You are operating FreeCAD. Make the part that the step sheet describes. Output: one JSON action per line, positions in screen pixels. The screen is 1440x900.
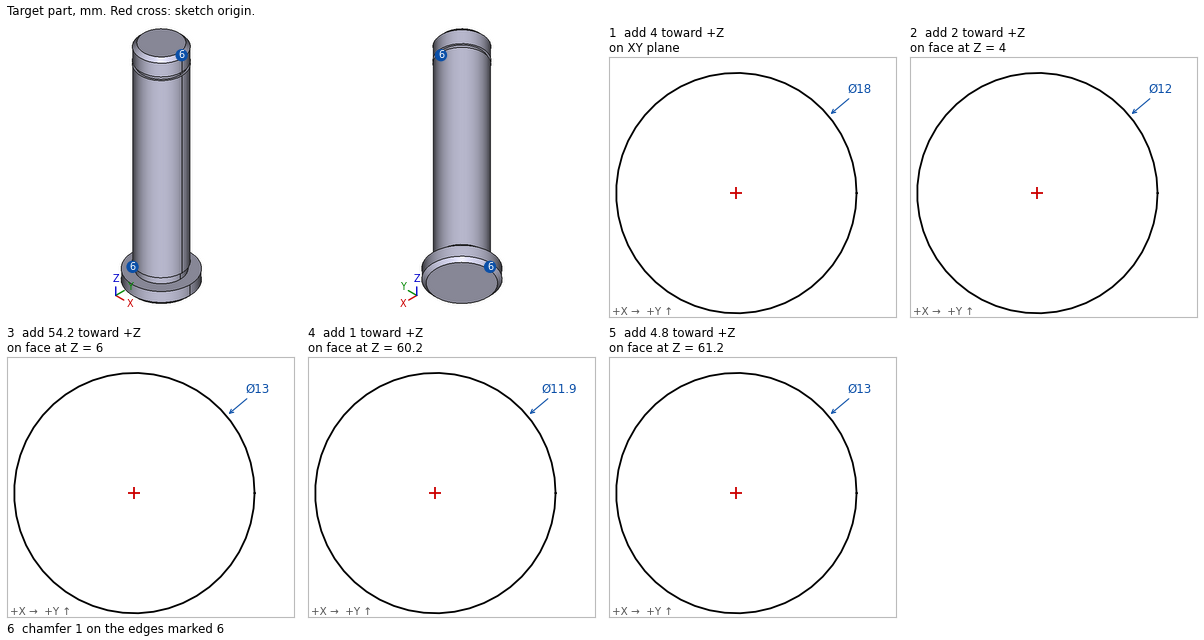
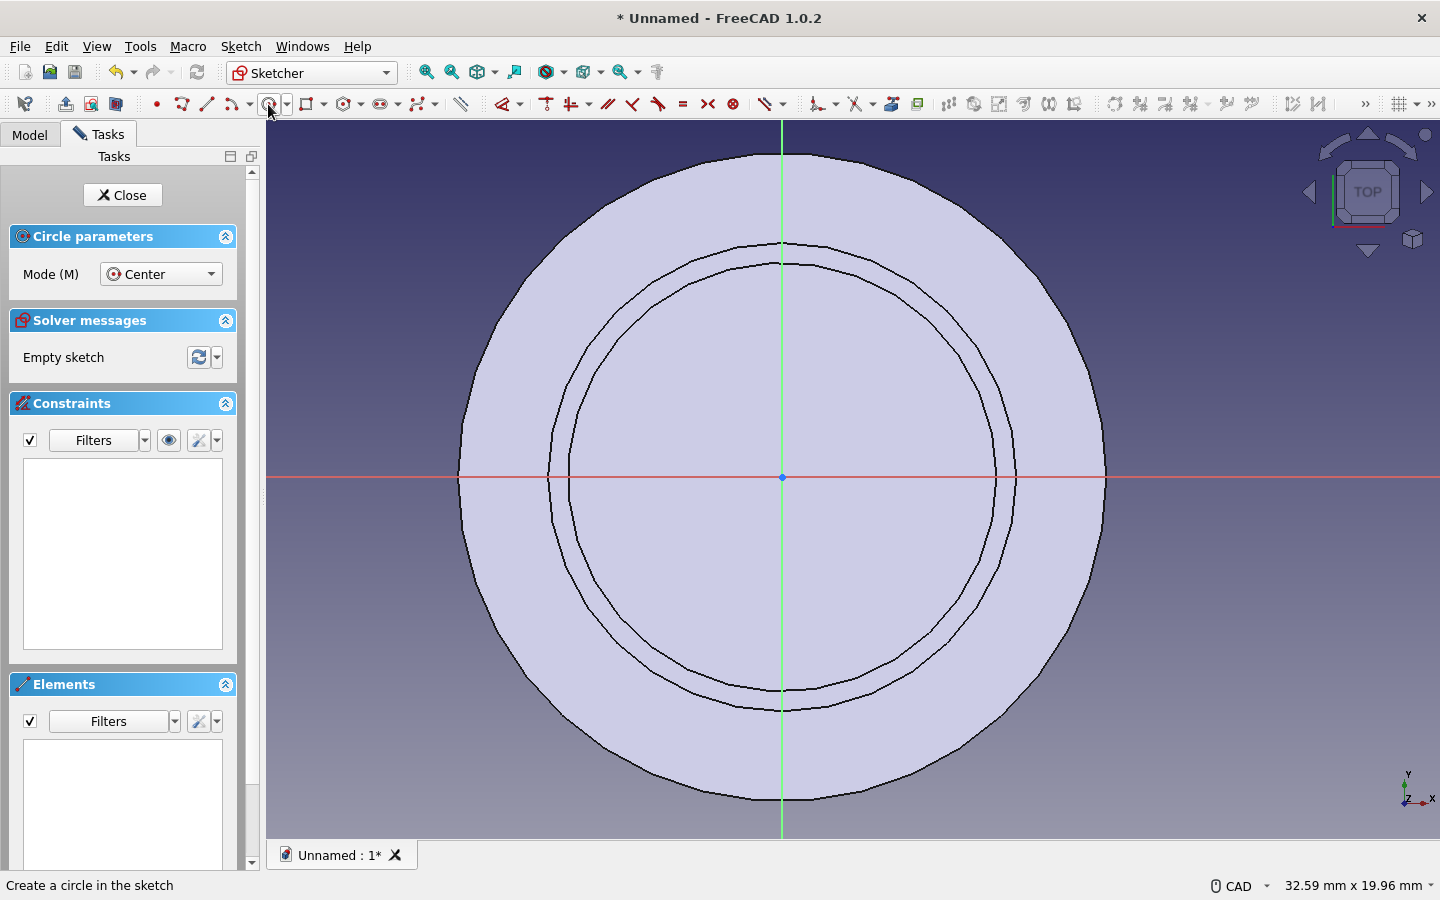
{"action": "left_click", "coordinate": [782, 477]}
{"action": "left_click", "coordinate": [948, 312]}
{"action": "key", "text": "Escape"}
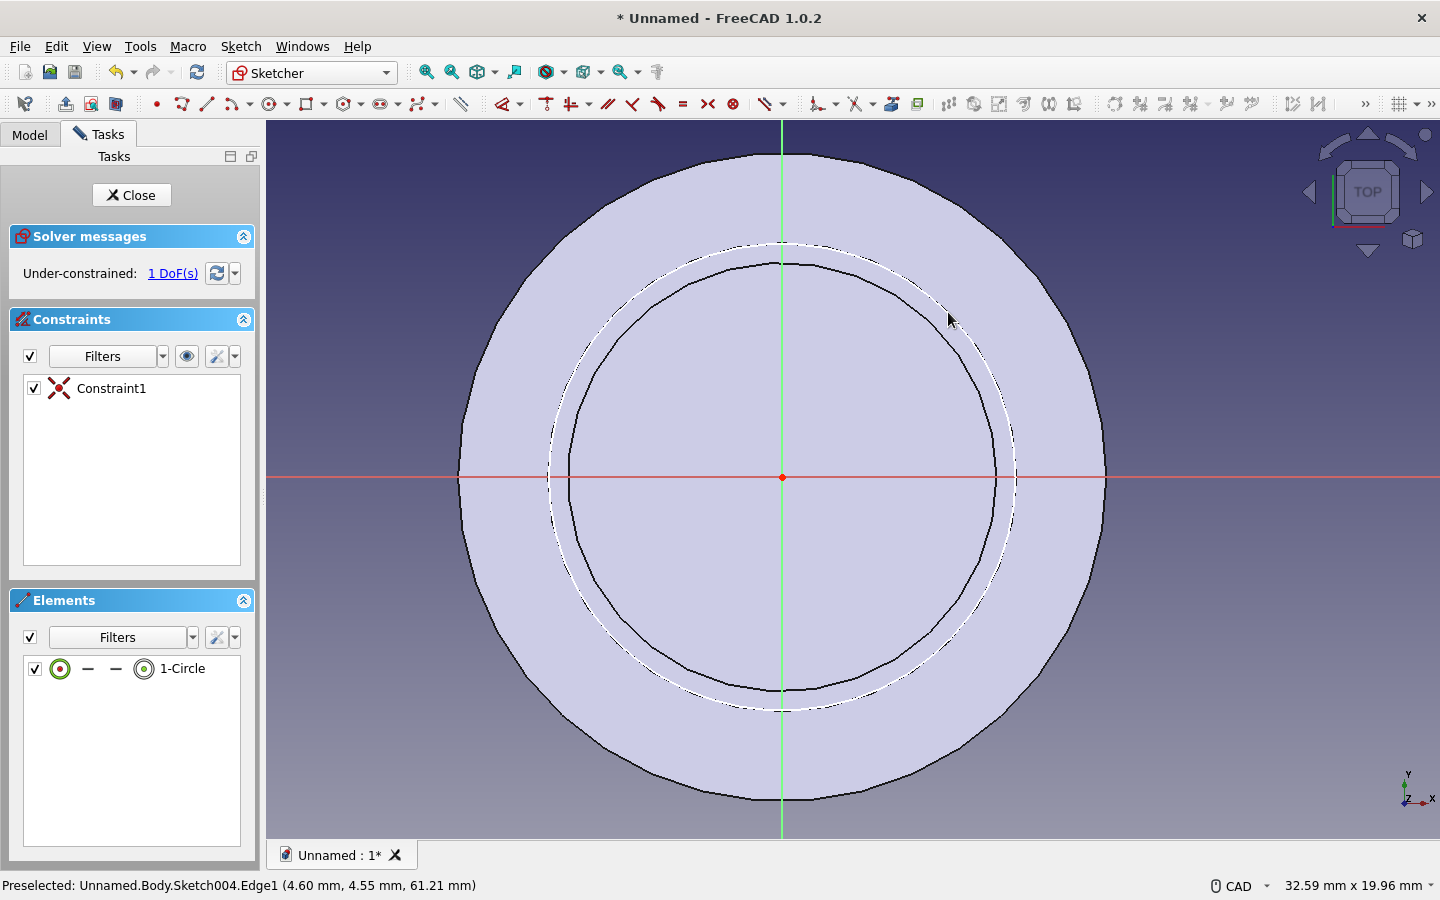
{"action": "left_click", "coordinate": [502, 104]}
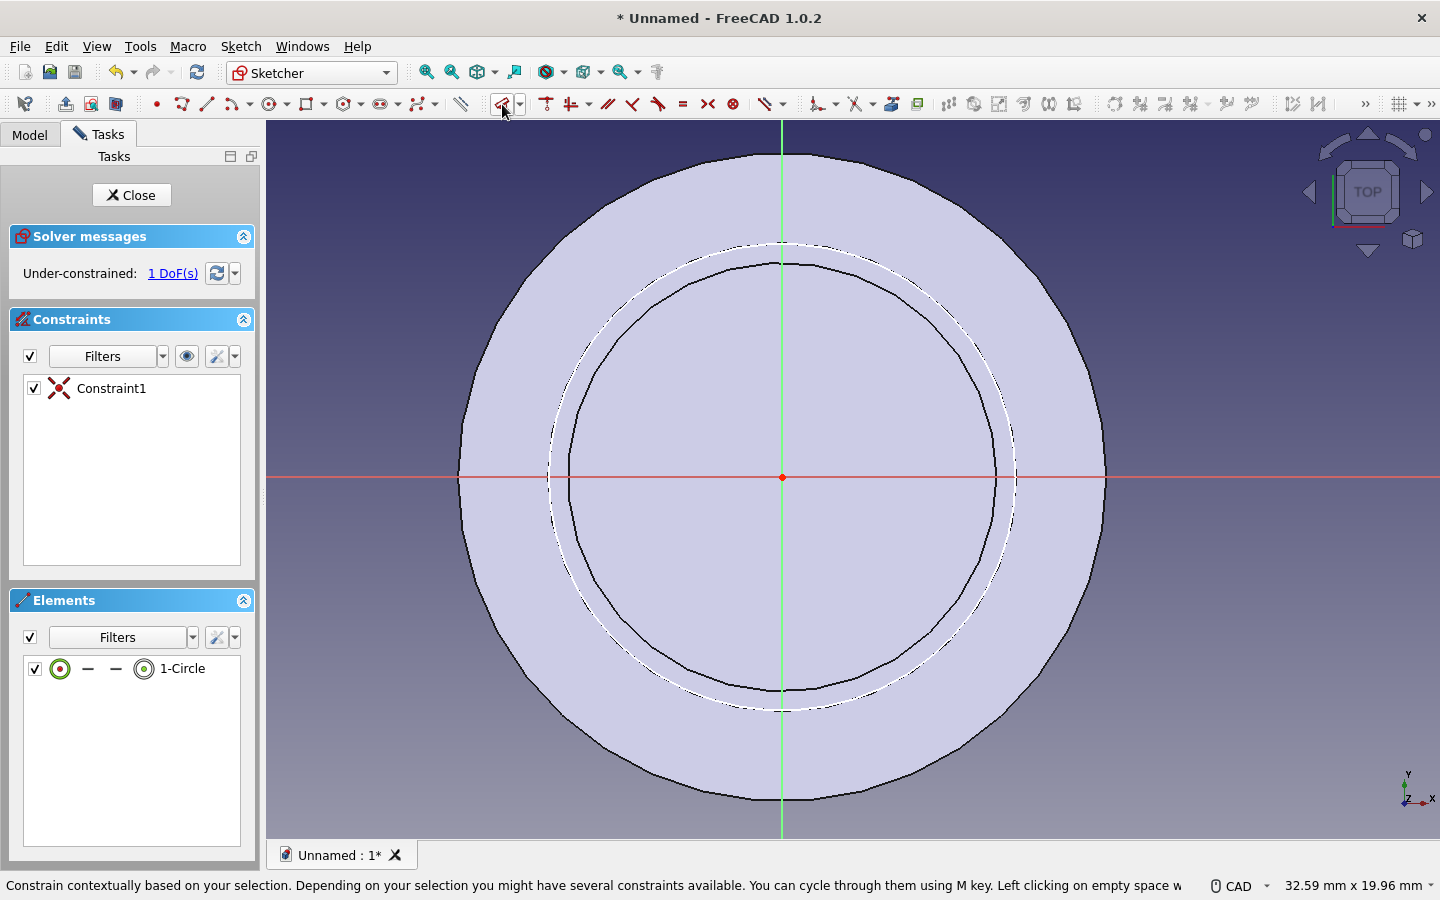
{"action": "left_click", "coordinate": [947, 312]}
{"action": "left_click", "coordinate": [970, 289]}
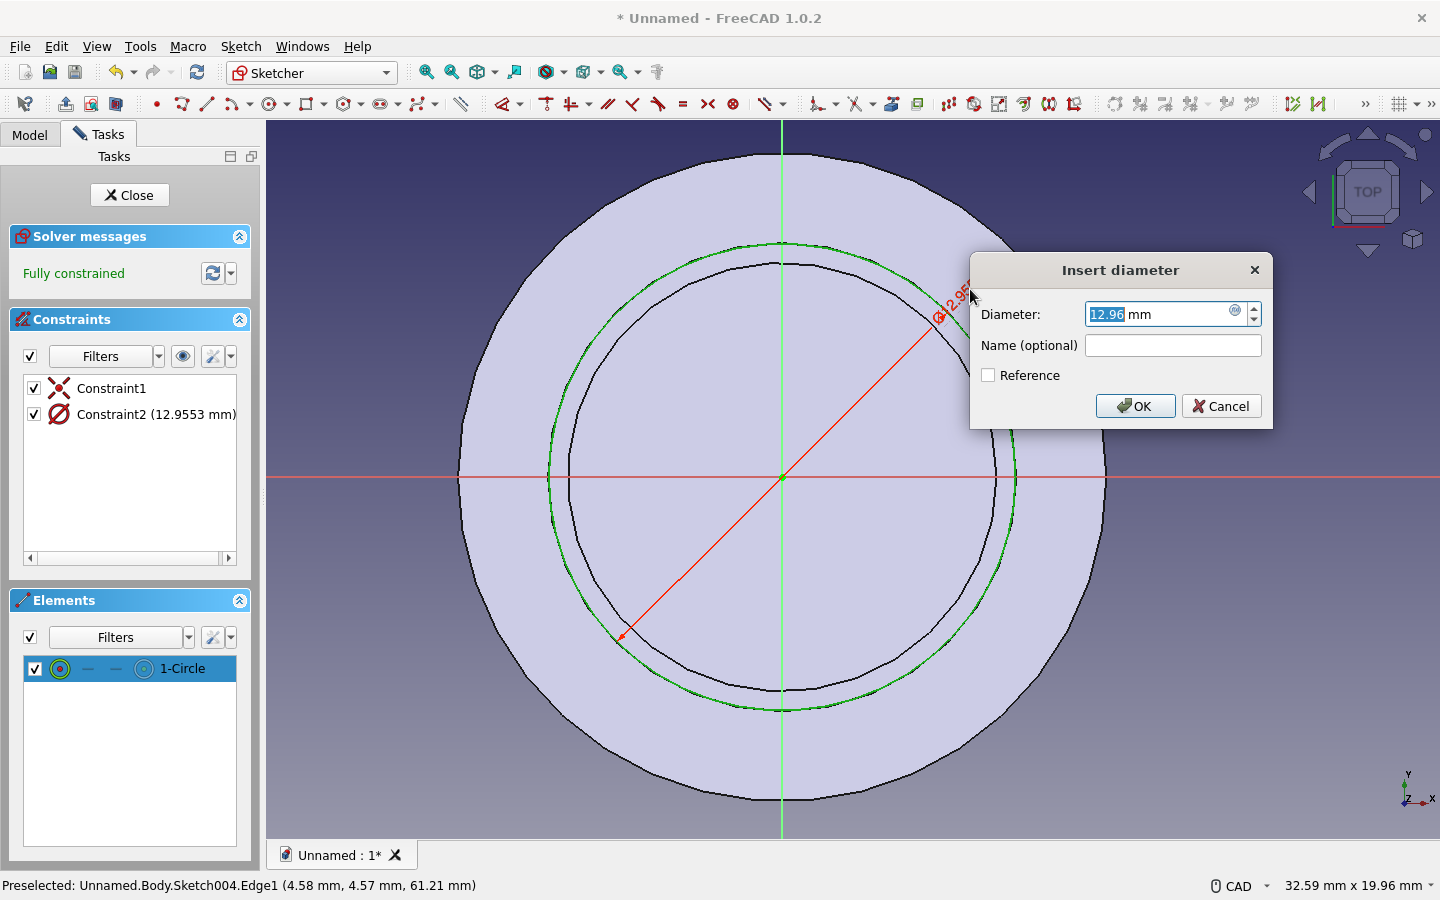
{"action": "type", "text": "13"}
{"action": "key", "text": "Return"}
{"action": "key", "text": "Escape"}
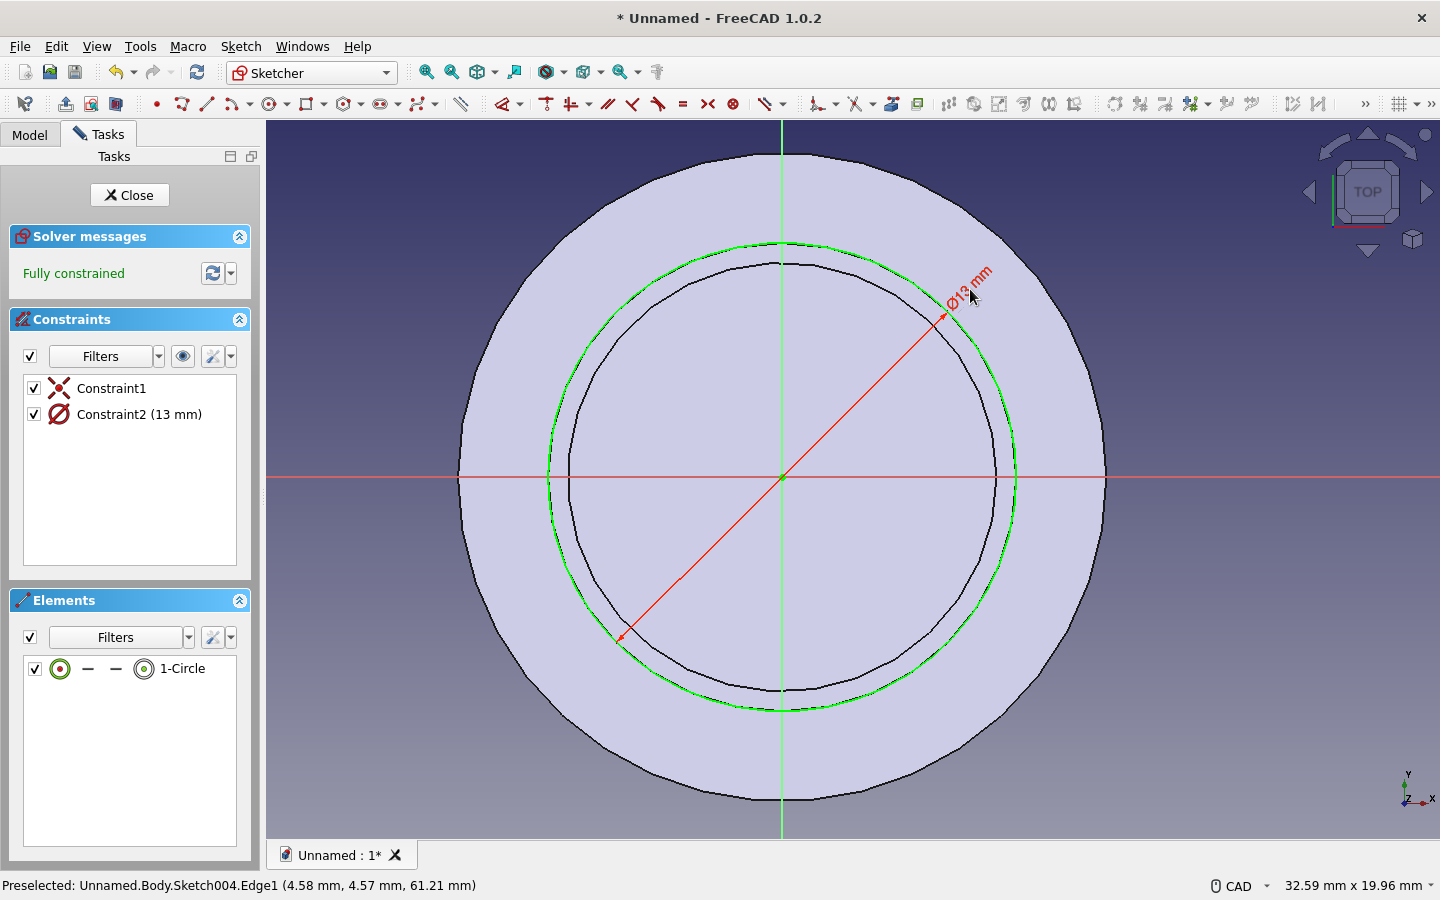
{"action": "left_click", "coordinate": [130, 195]}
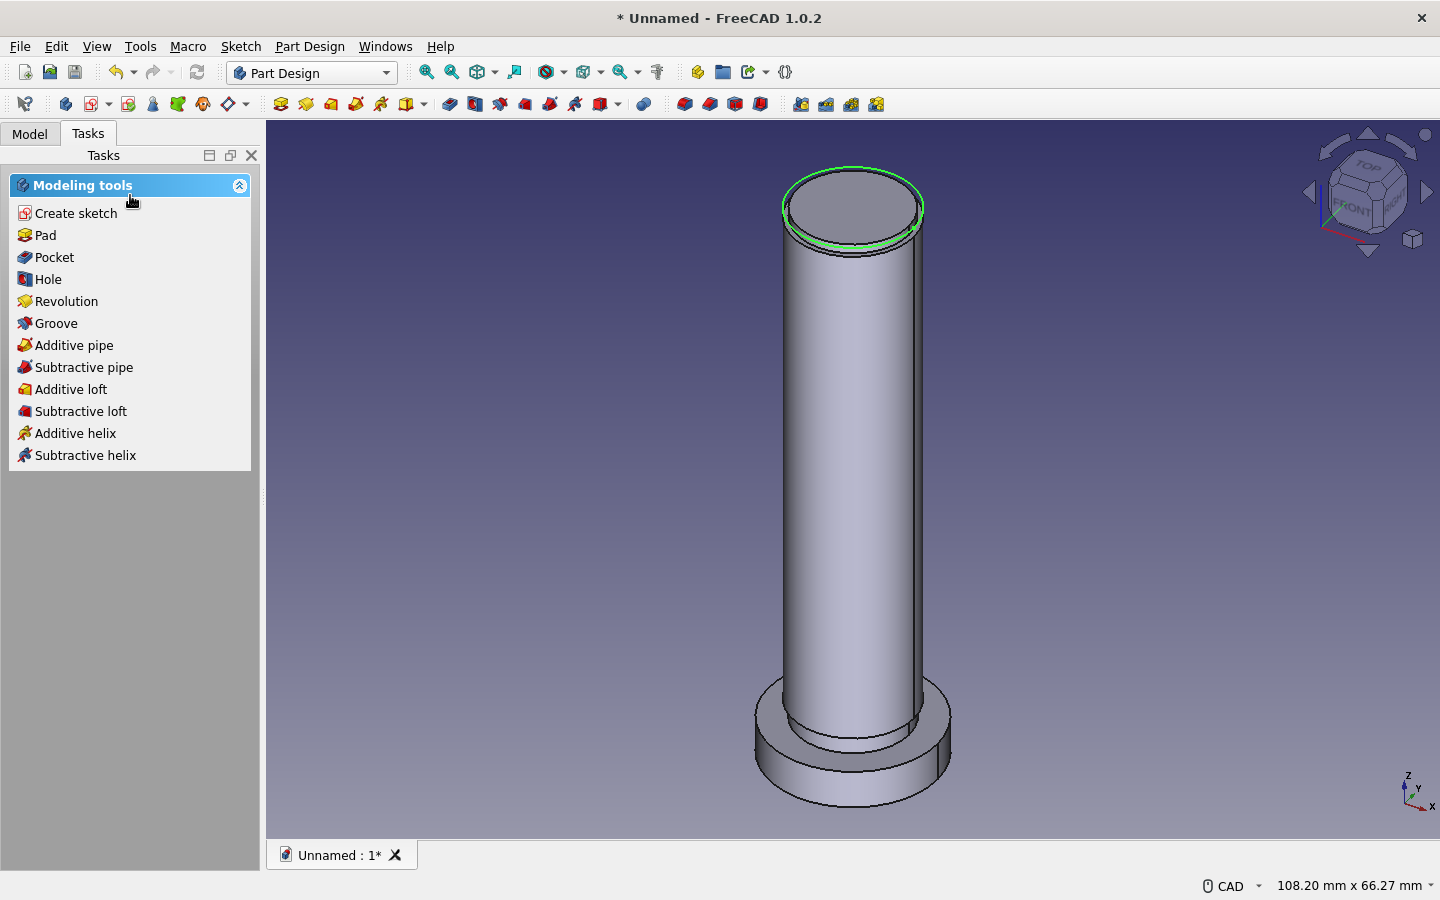
{"action": "left_click", "coordinate": [281, 104]}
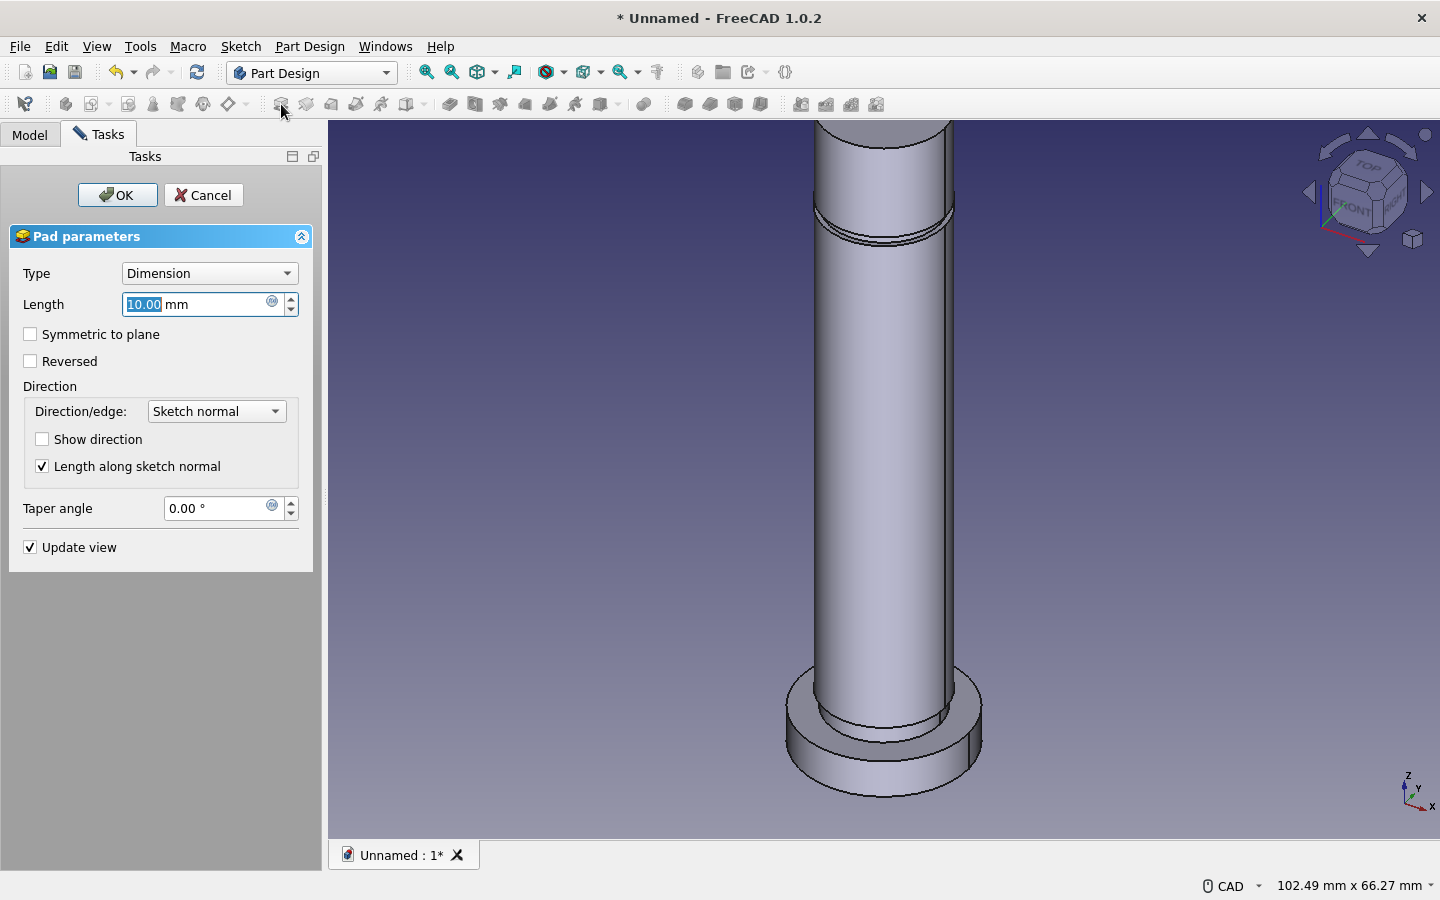
{"action": "type", "text": "4.8"}
{"action": "key", "text": "Tab"}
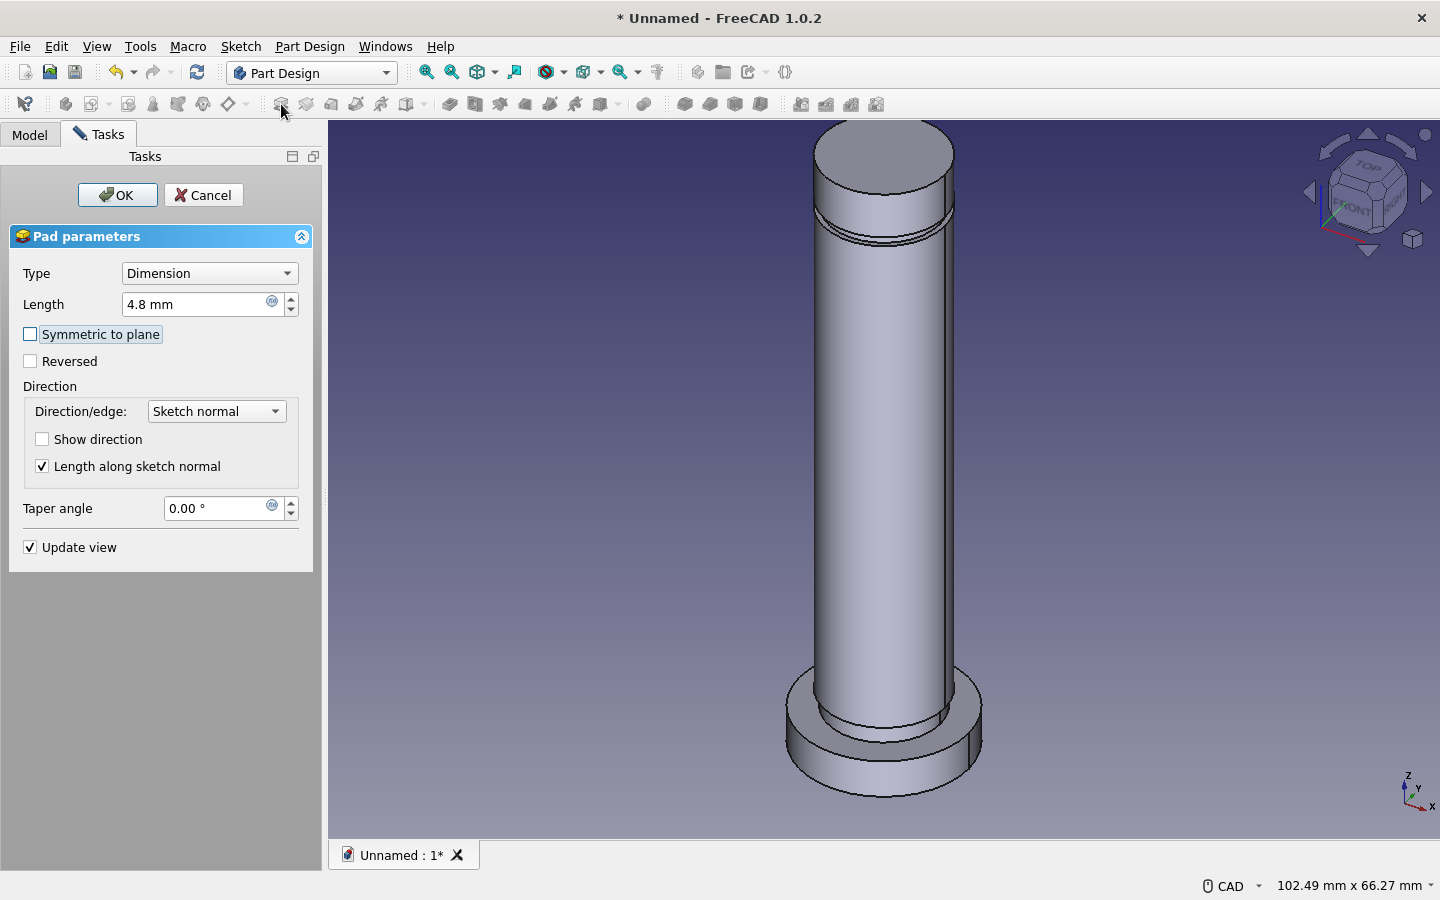
{"action": "left_click", "coordinate": [118, 195]}